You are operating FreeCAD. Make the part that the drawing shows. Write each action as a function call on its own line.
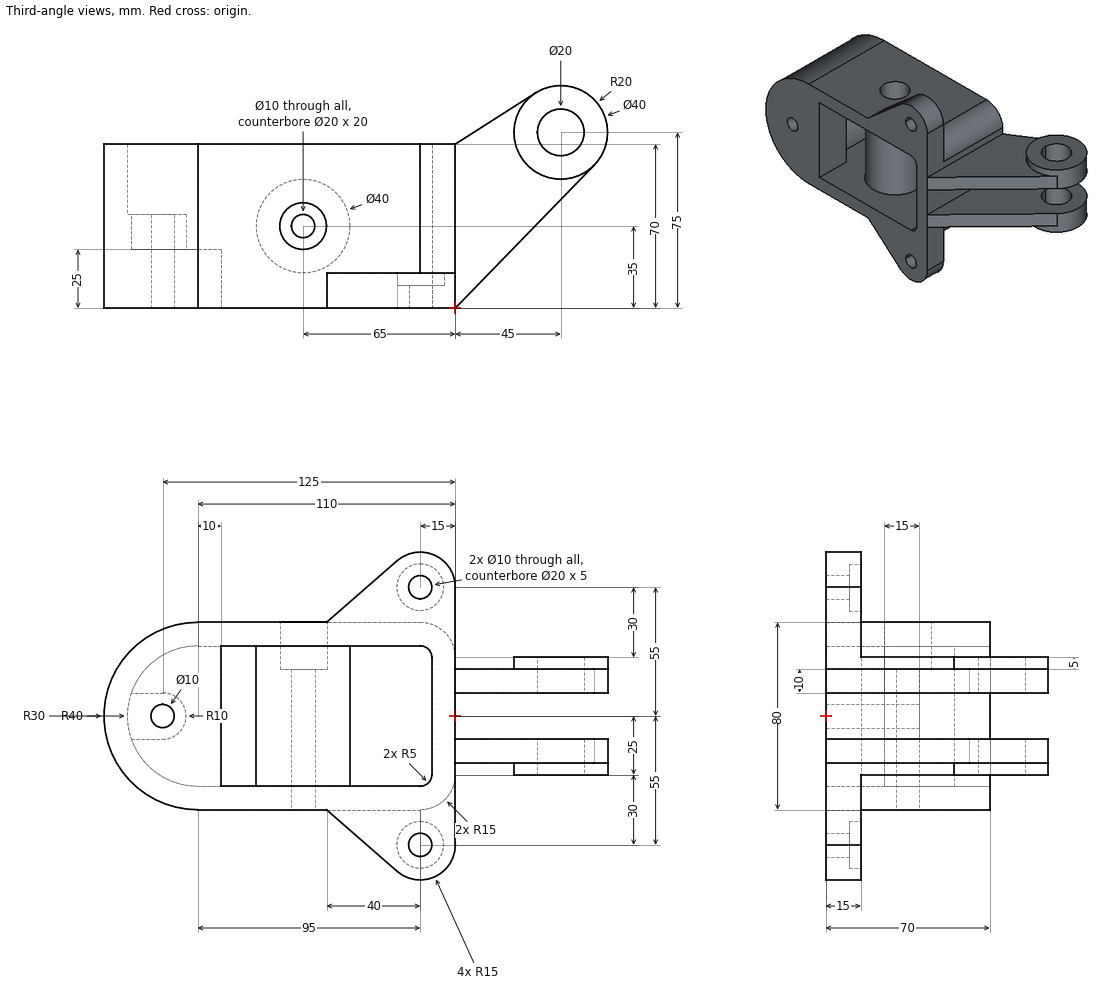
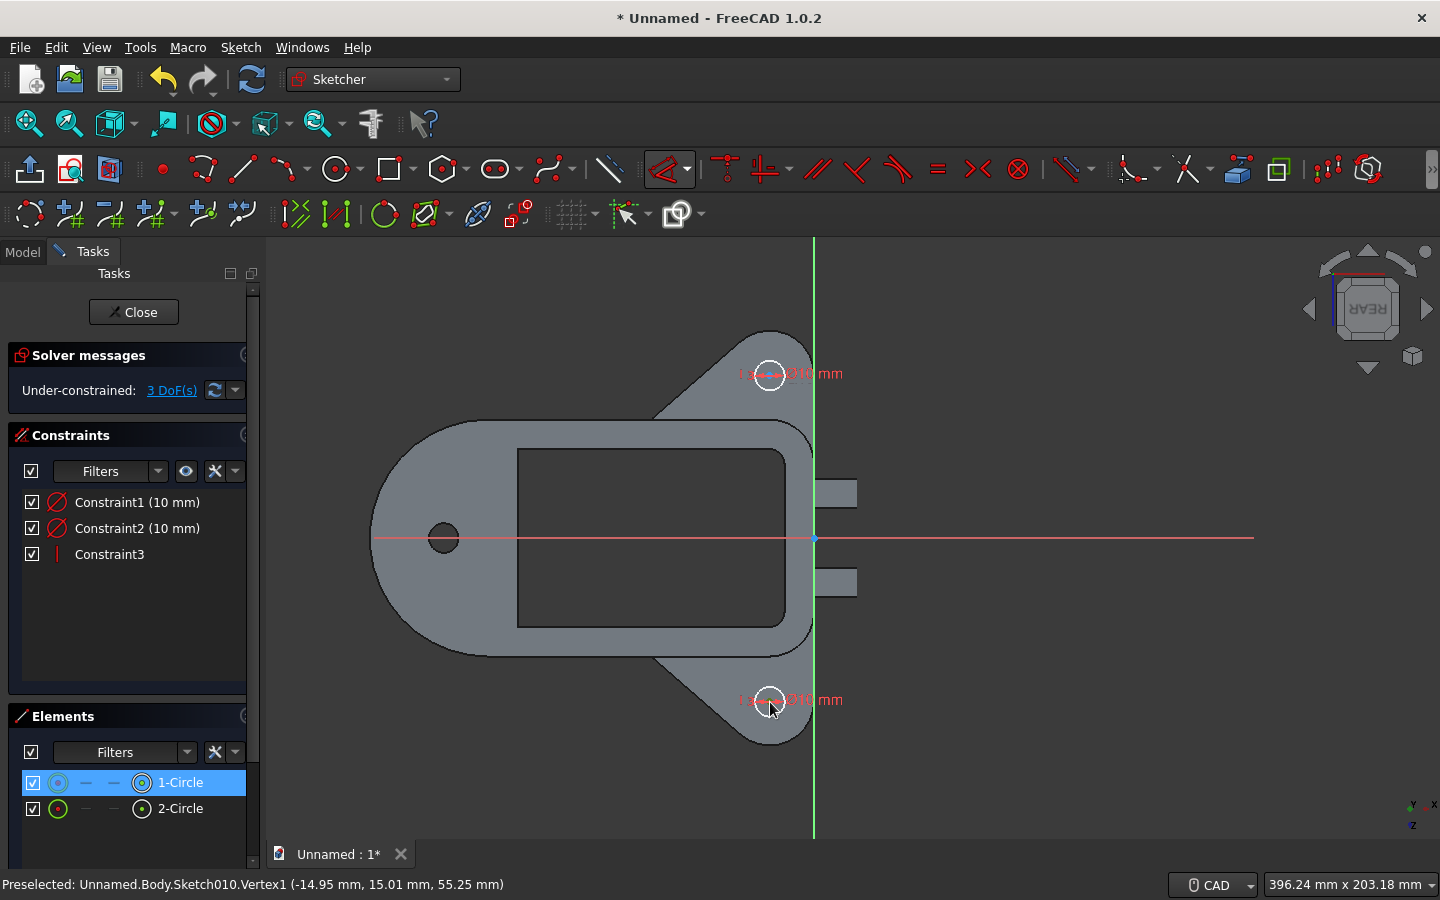
key(l)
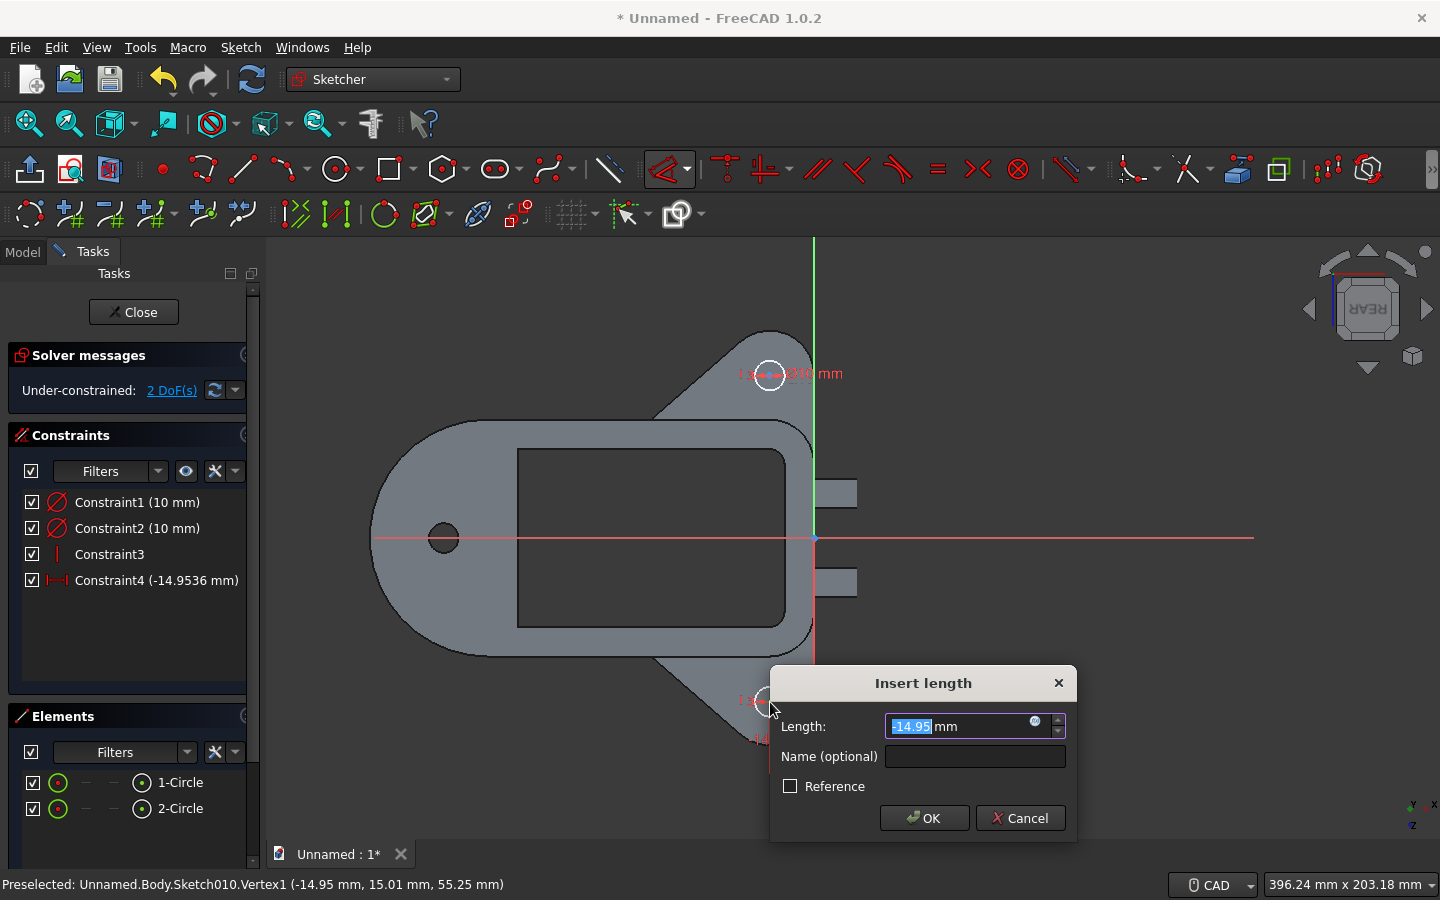
text(-15)
key(Return)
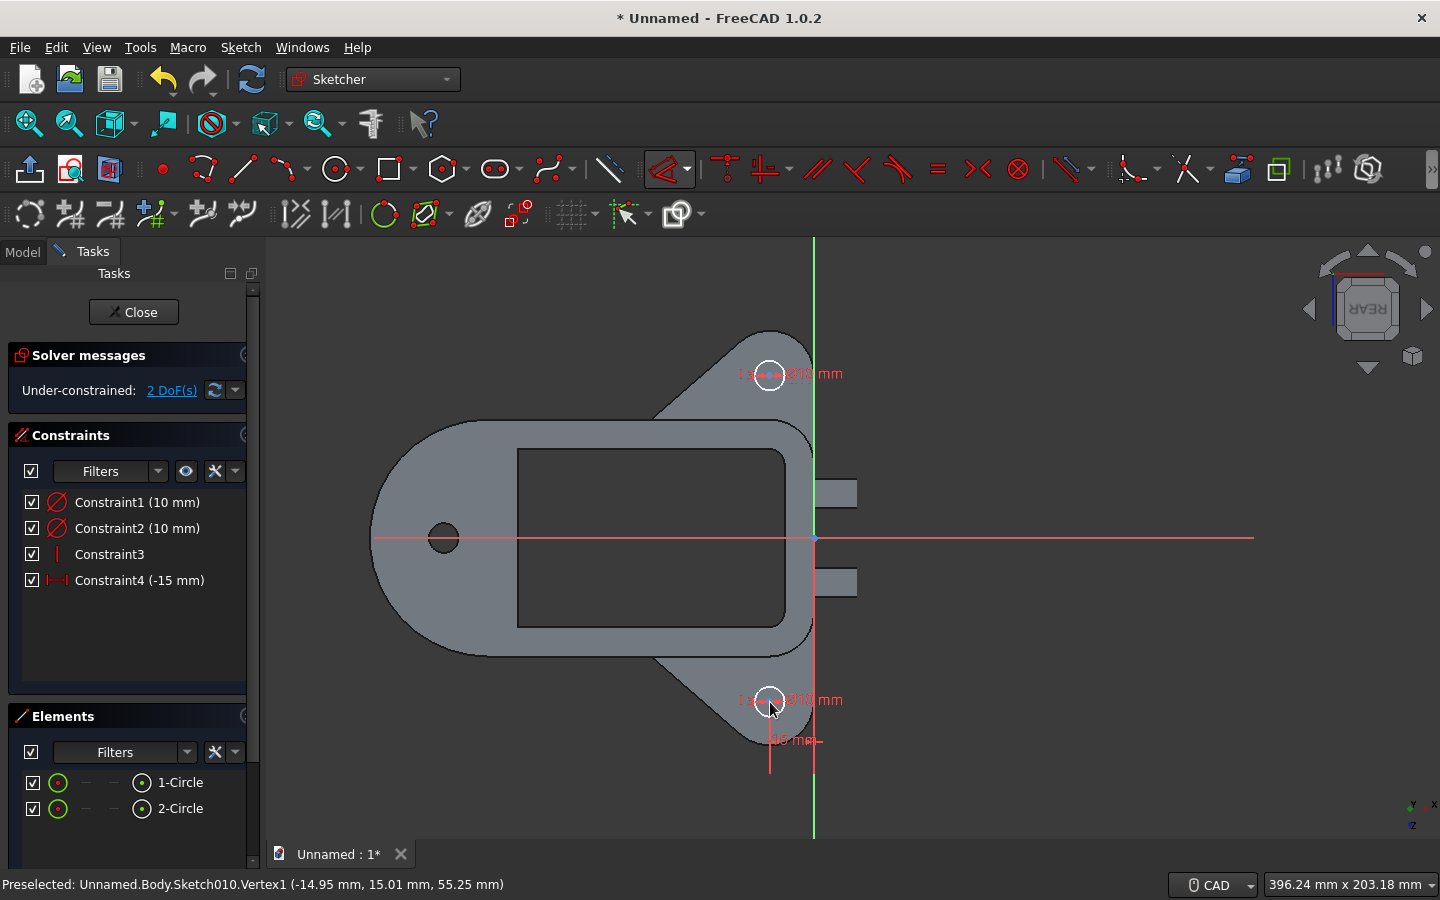
click(770, 702)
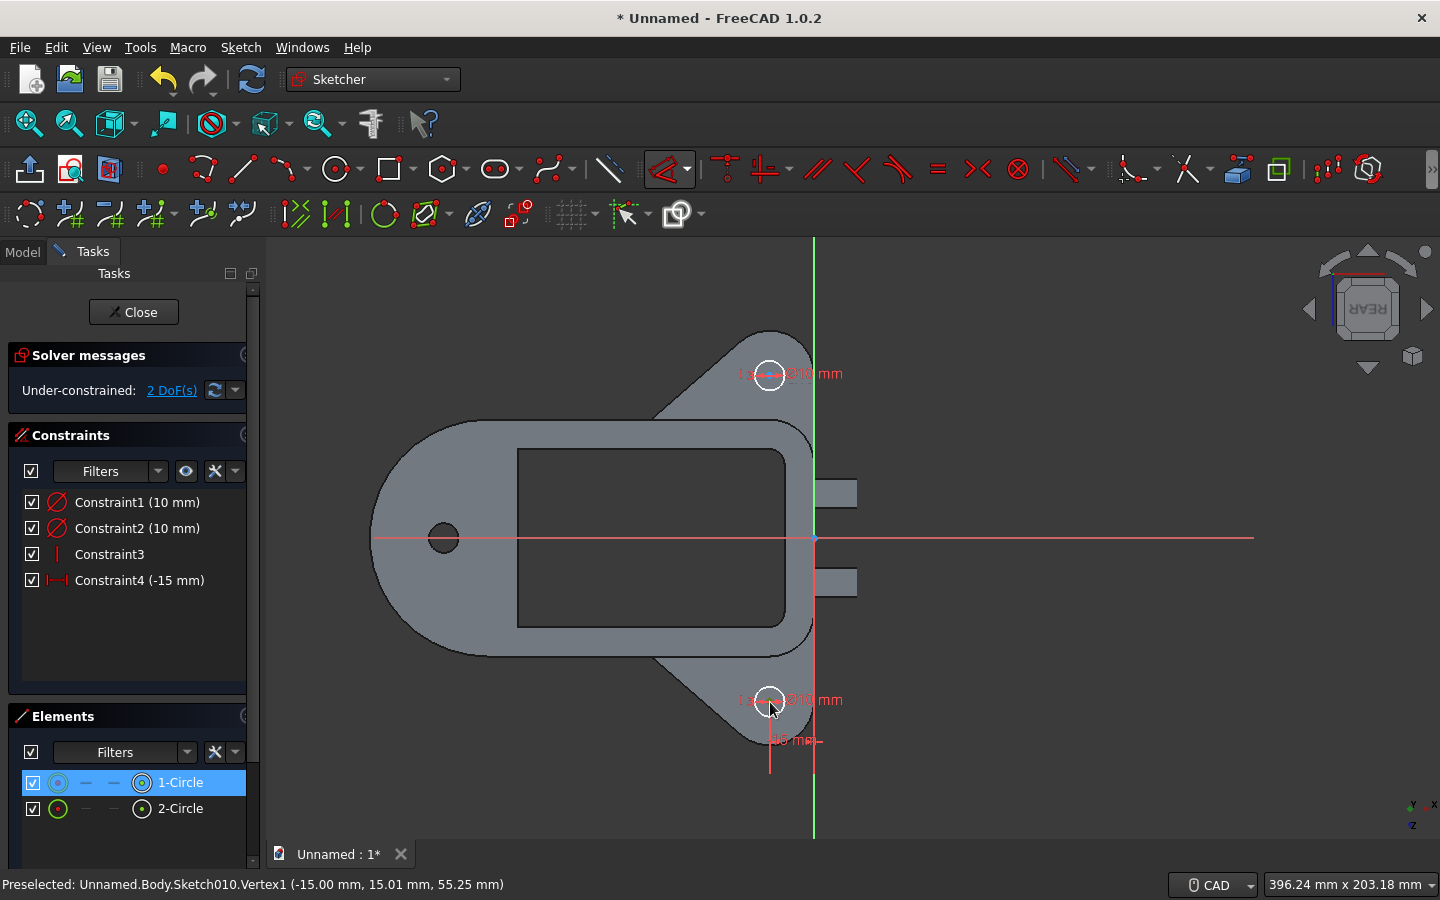
click(690, 170)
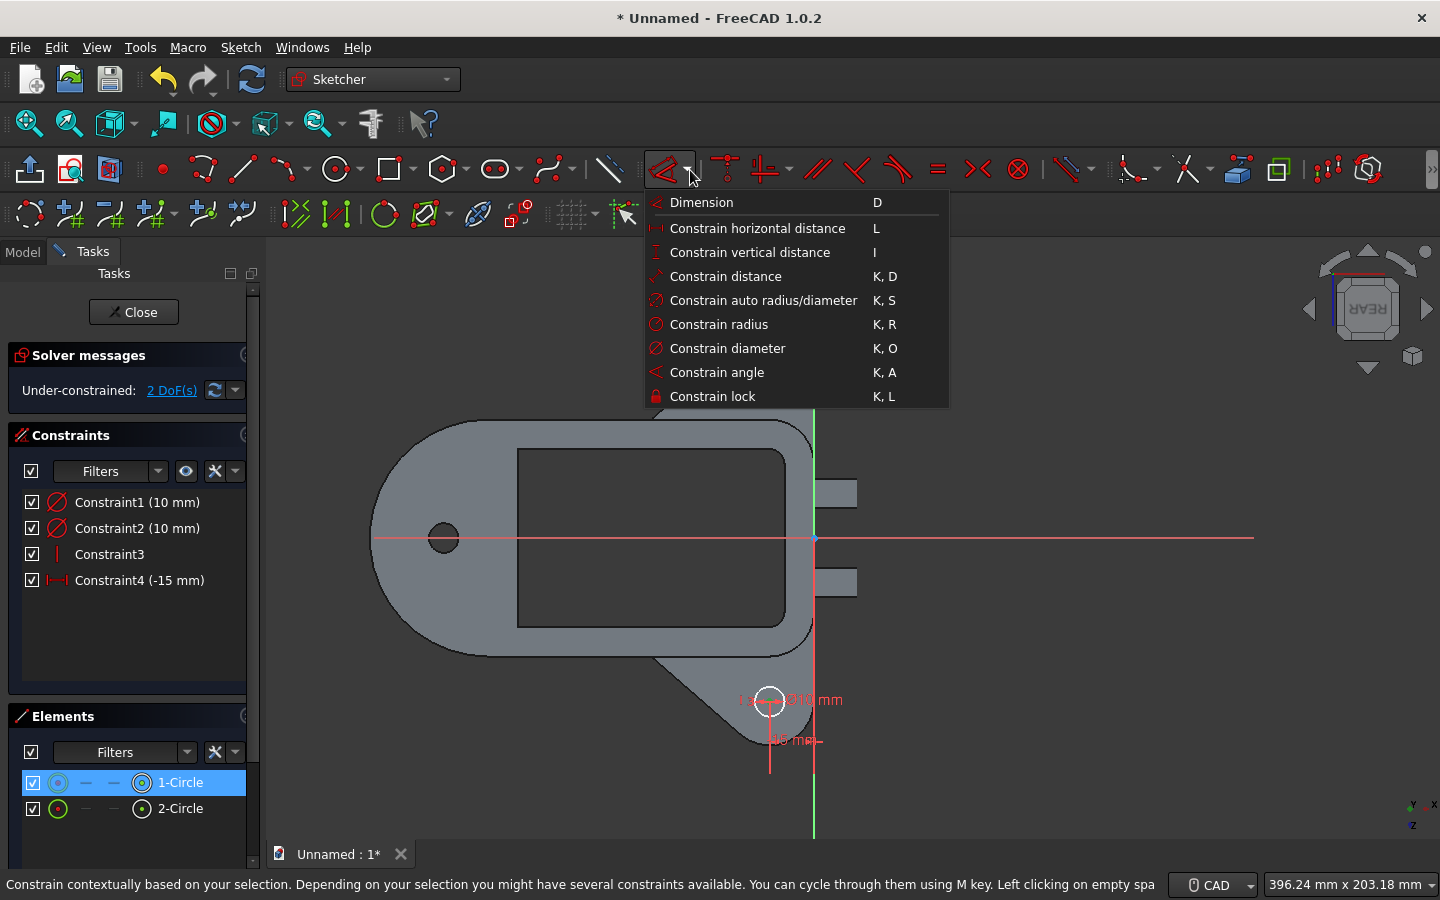
click(797, 252)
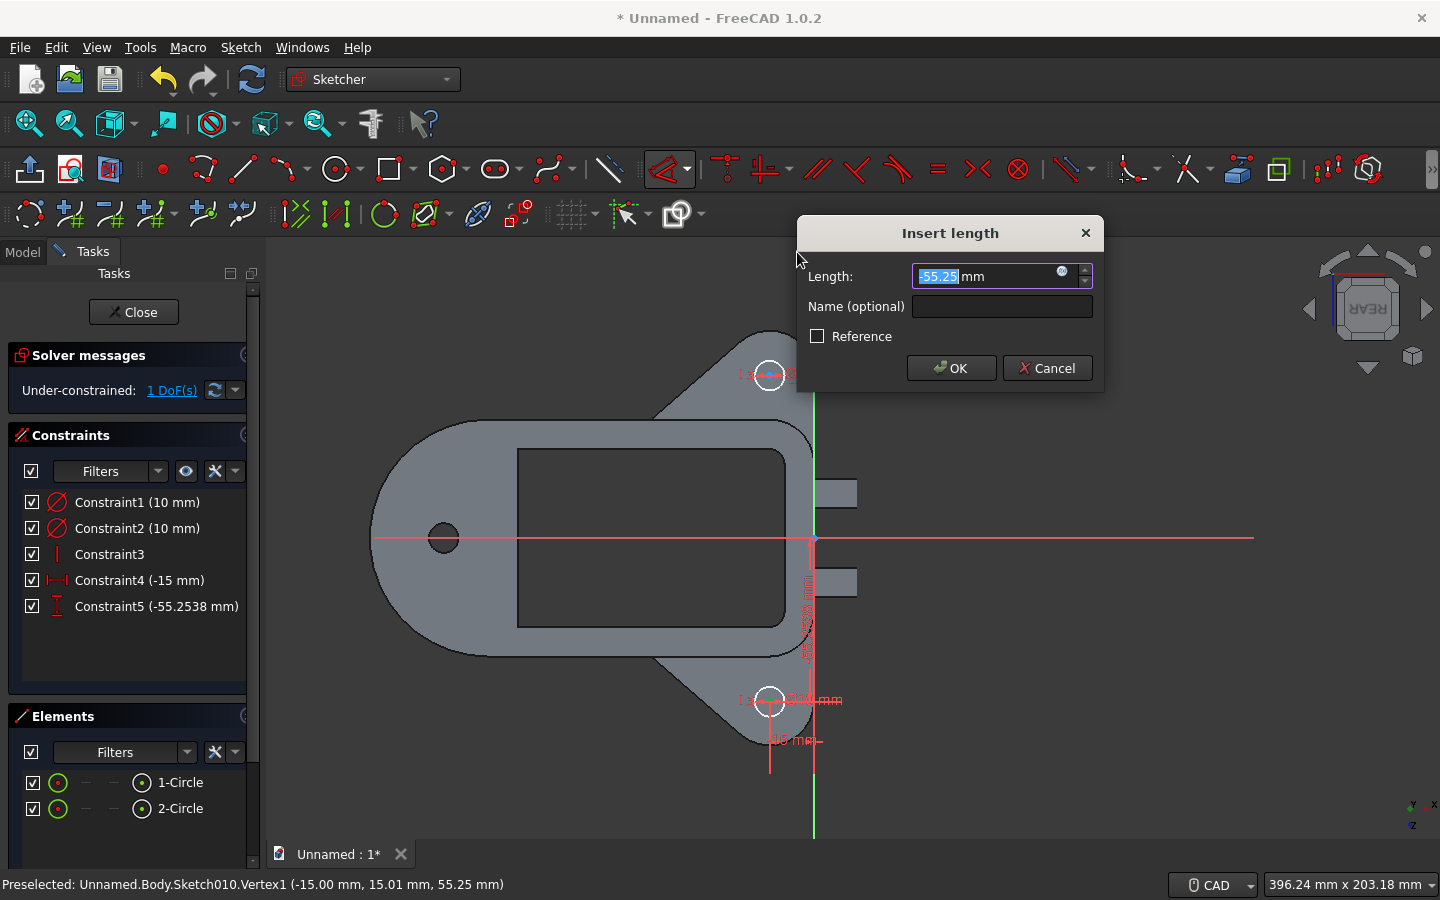
text(-55)
key(Return)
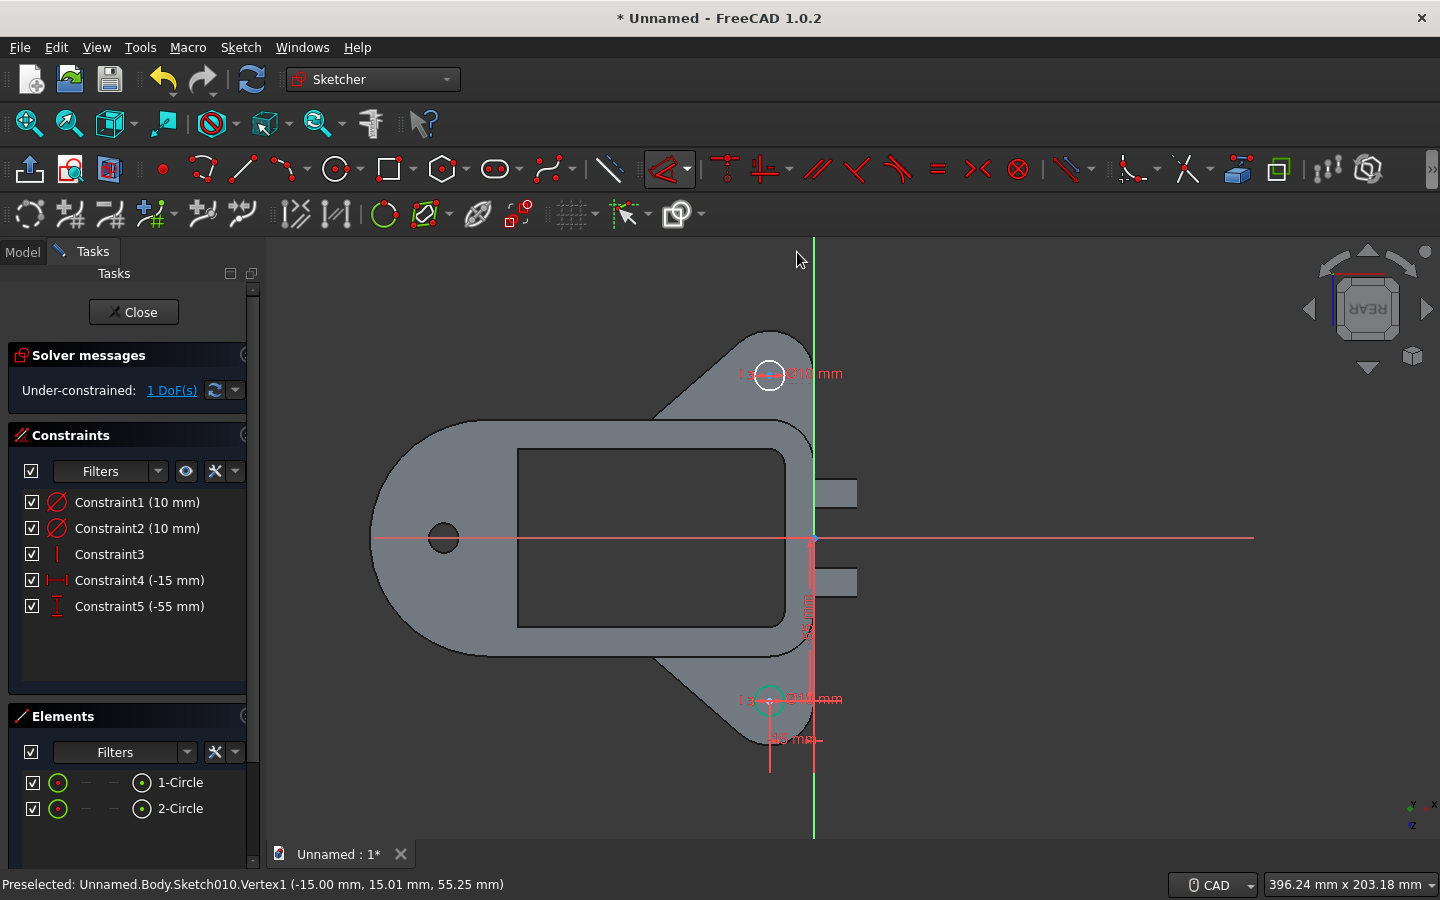
click(770, 376)